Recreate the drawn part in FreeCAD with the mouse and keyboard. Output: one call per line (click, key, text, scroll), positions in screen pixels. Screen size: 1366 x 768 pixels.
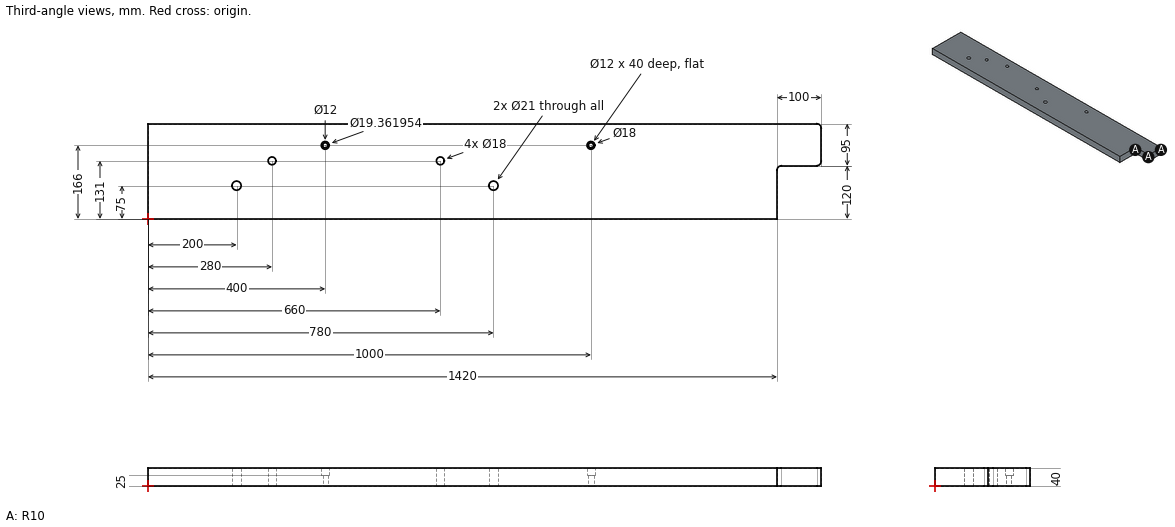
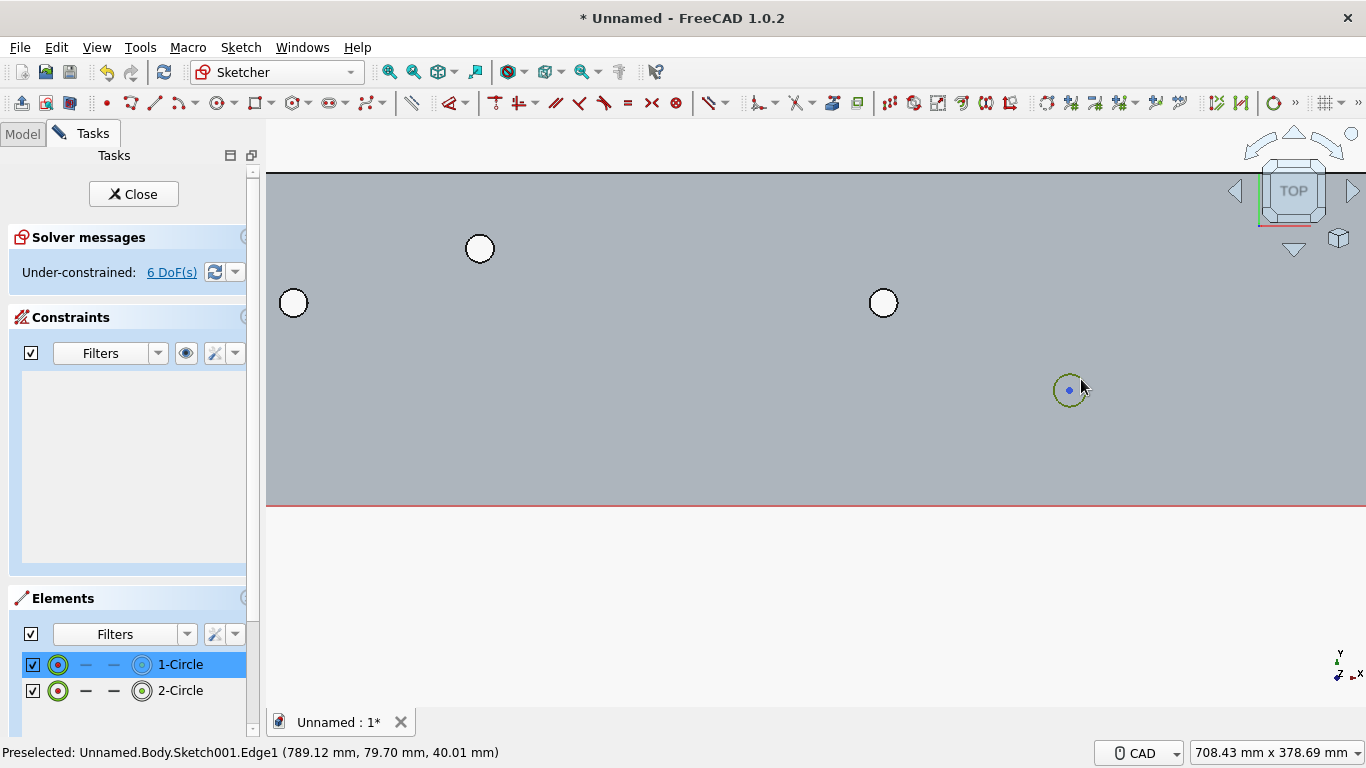
scroll(1082, 380, down, 3)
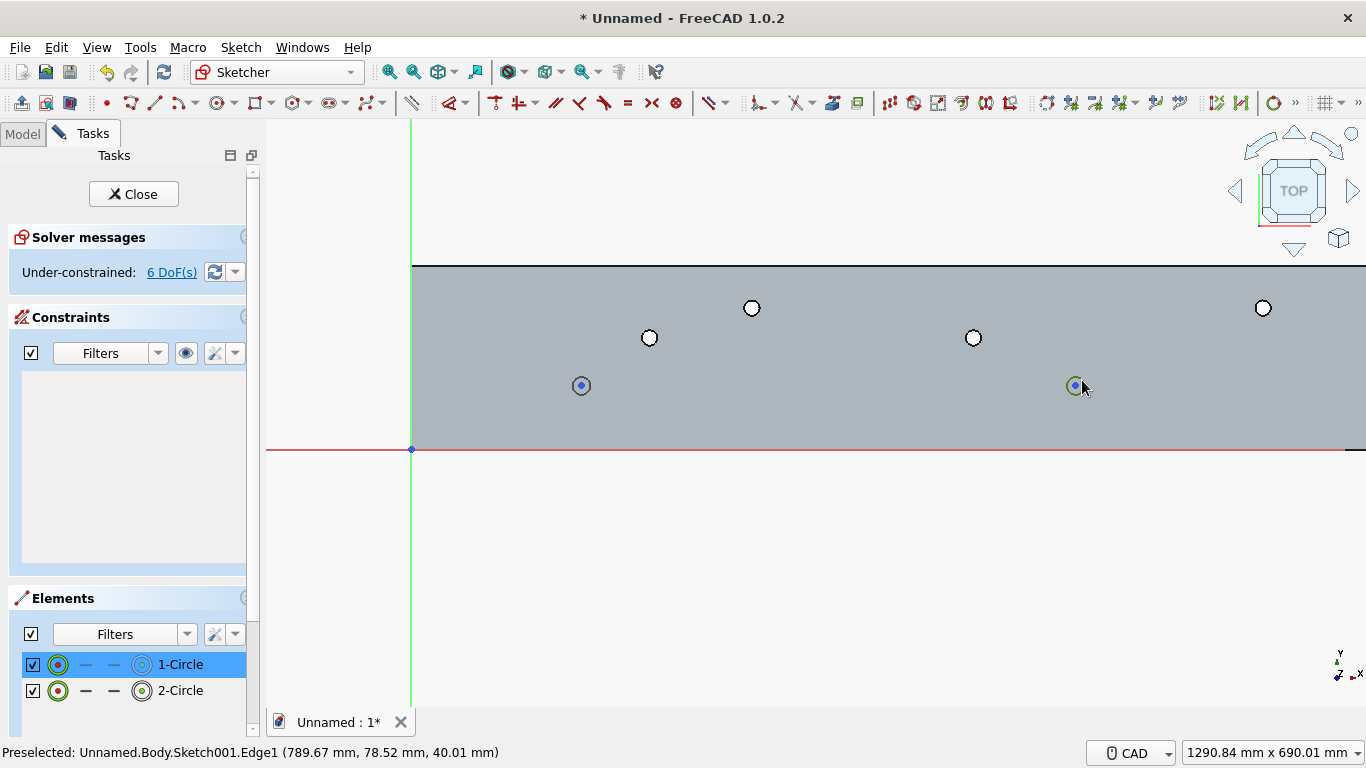
scroll(588, 380, up, 3)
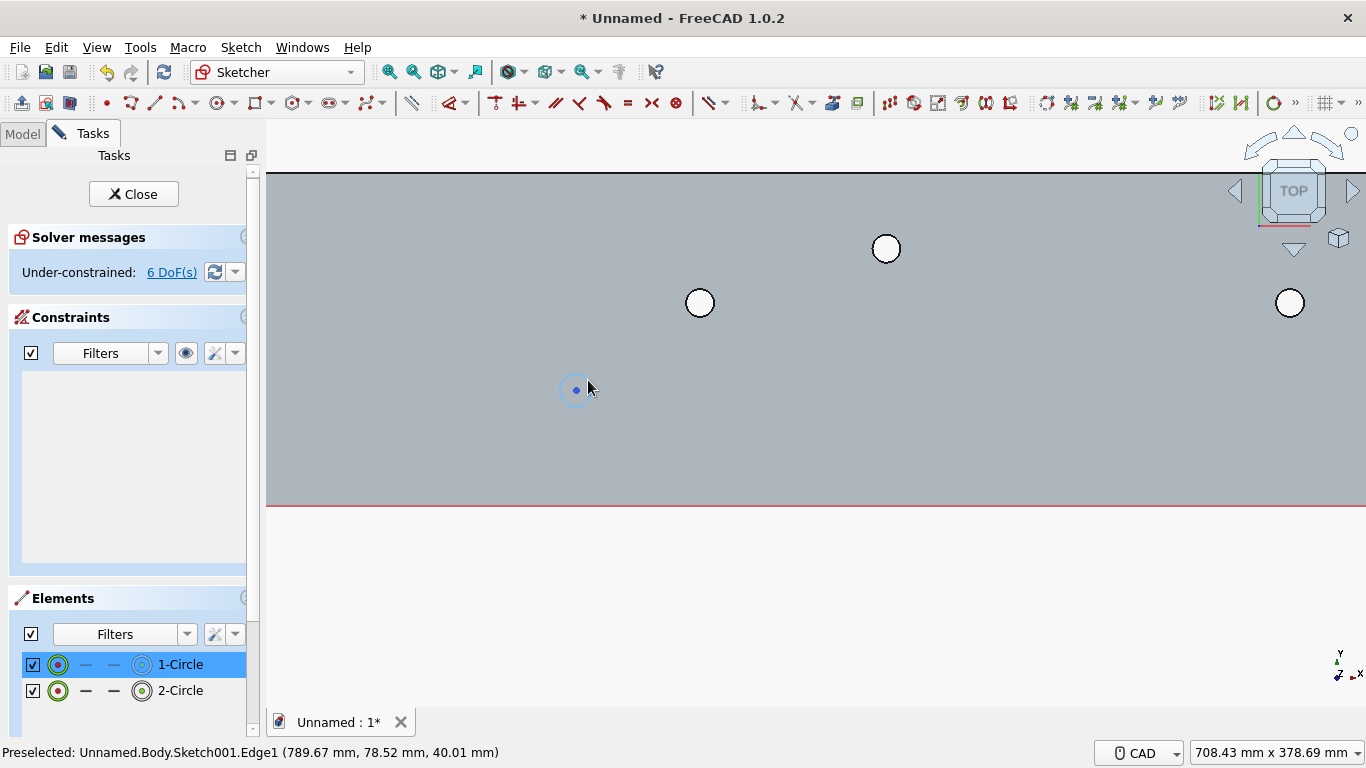
click(587, 379)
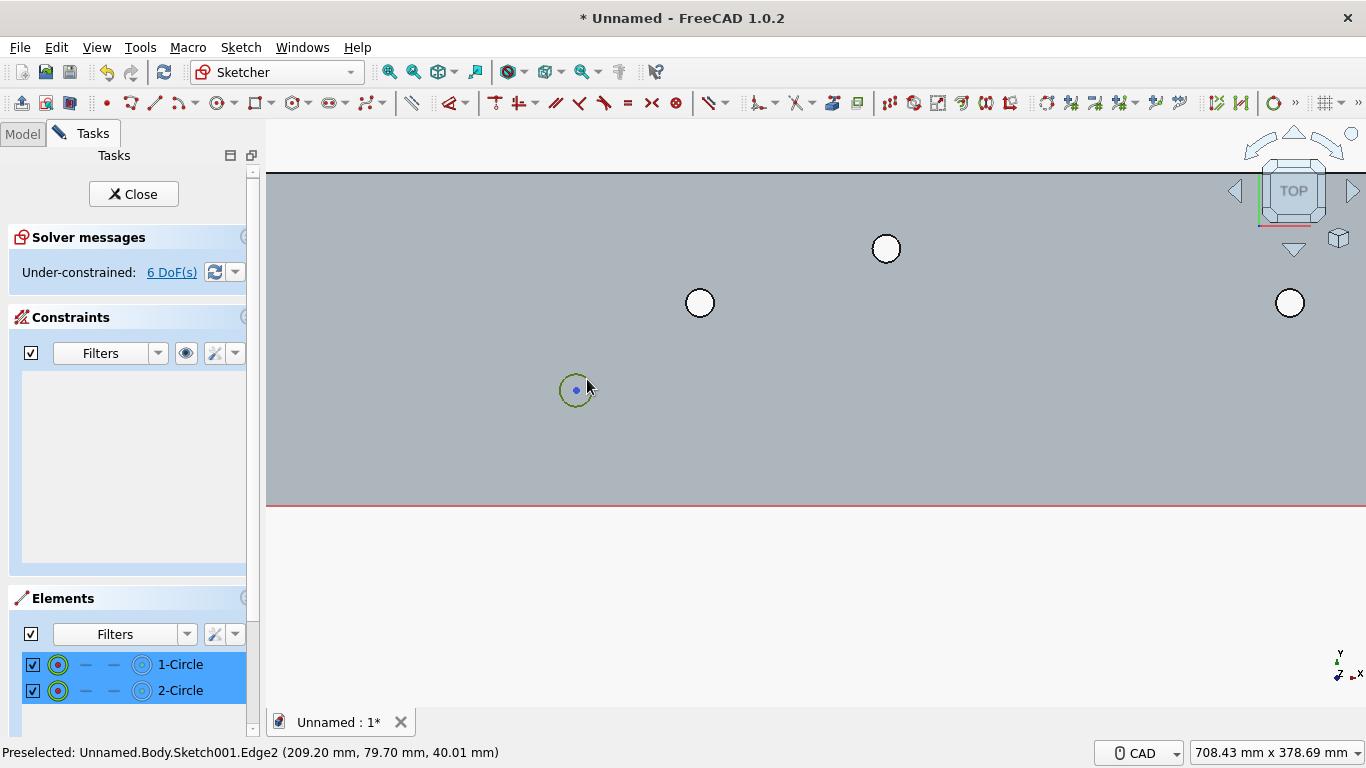
key(e)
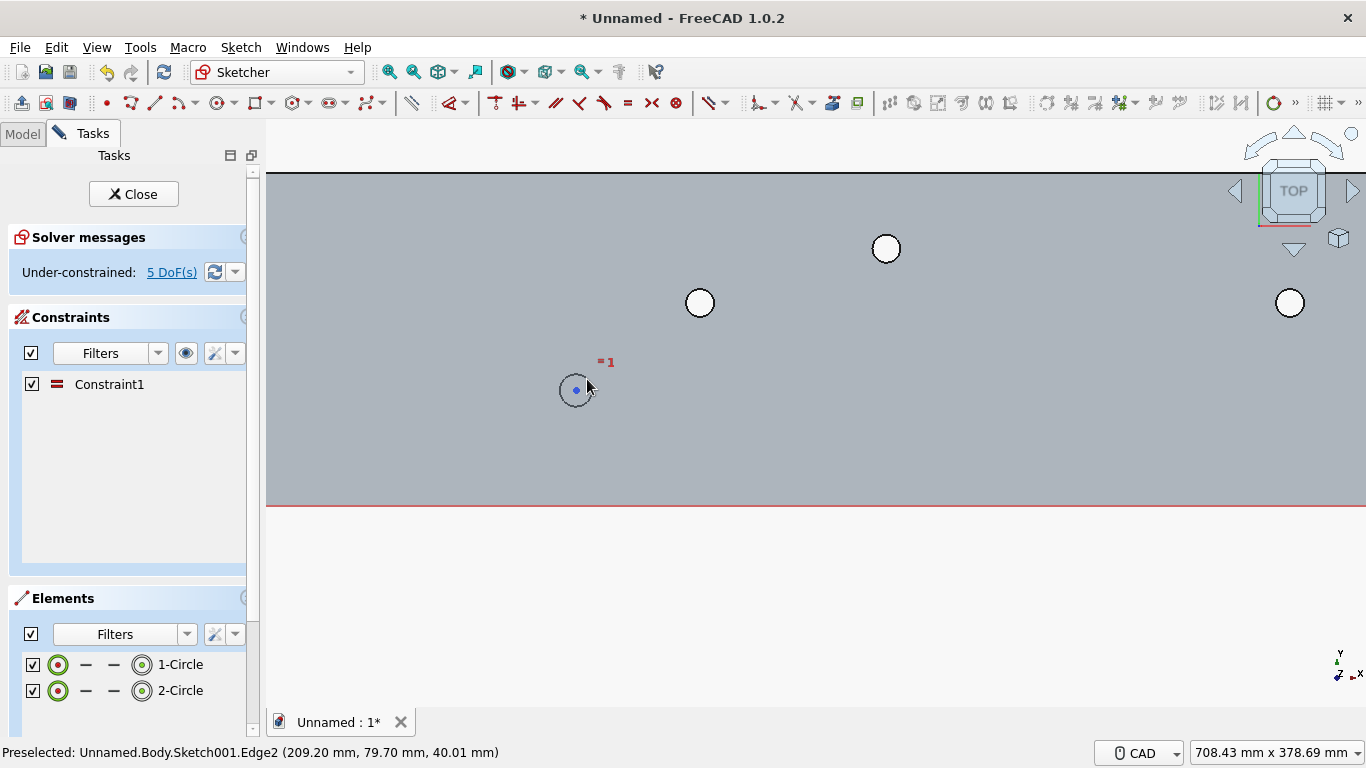
click(450, 104)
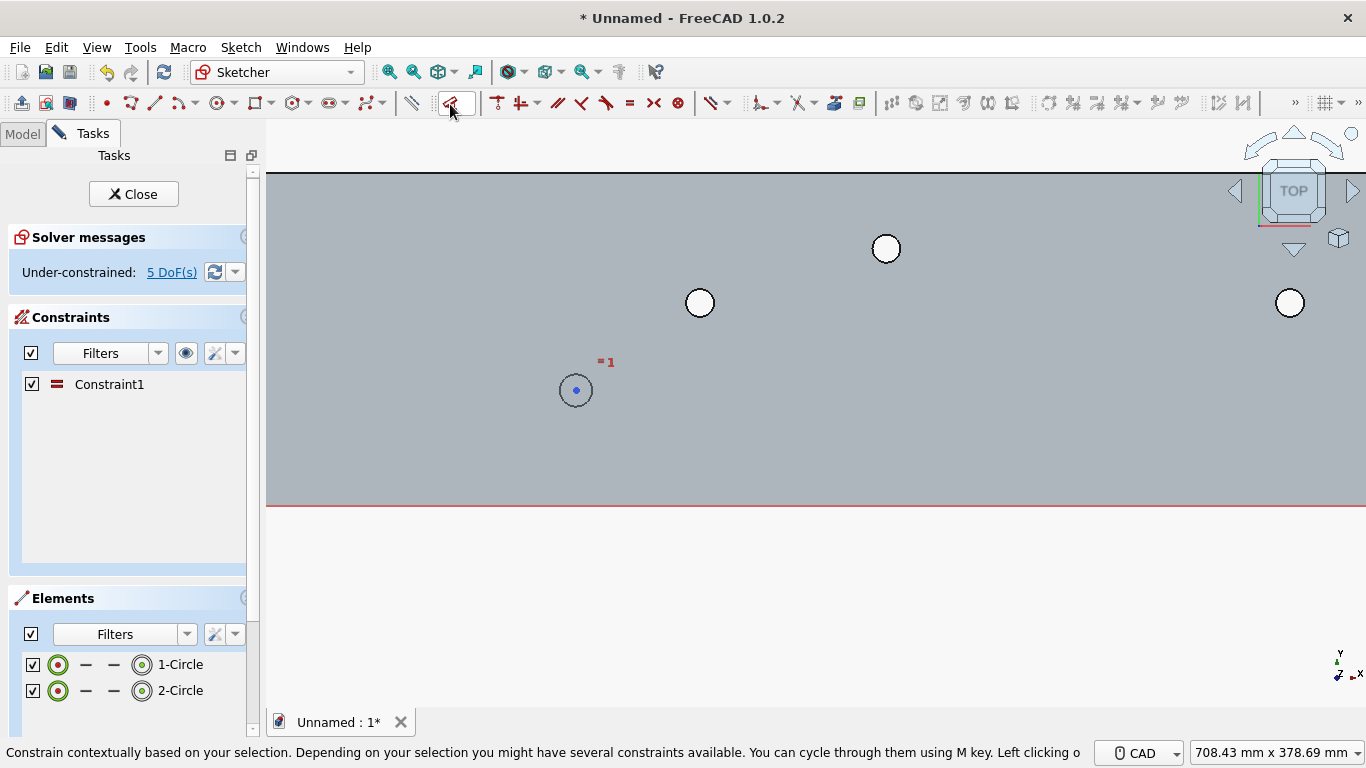
scroll(588, 380, down, 3)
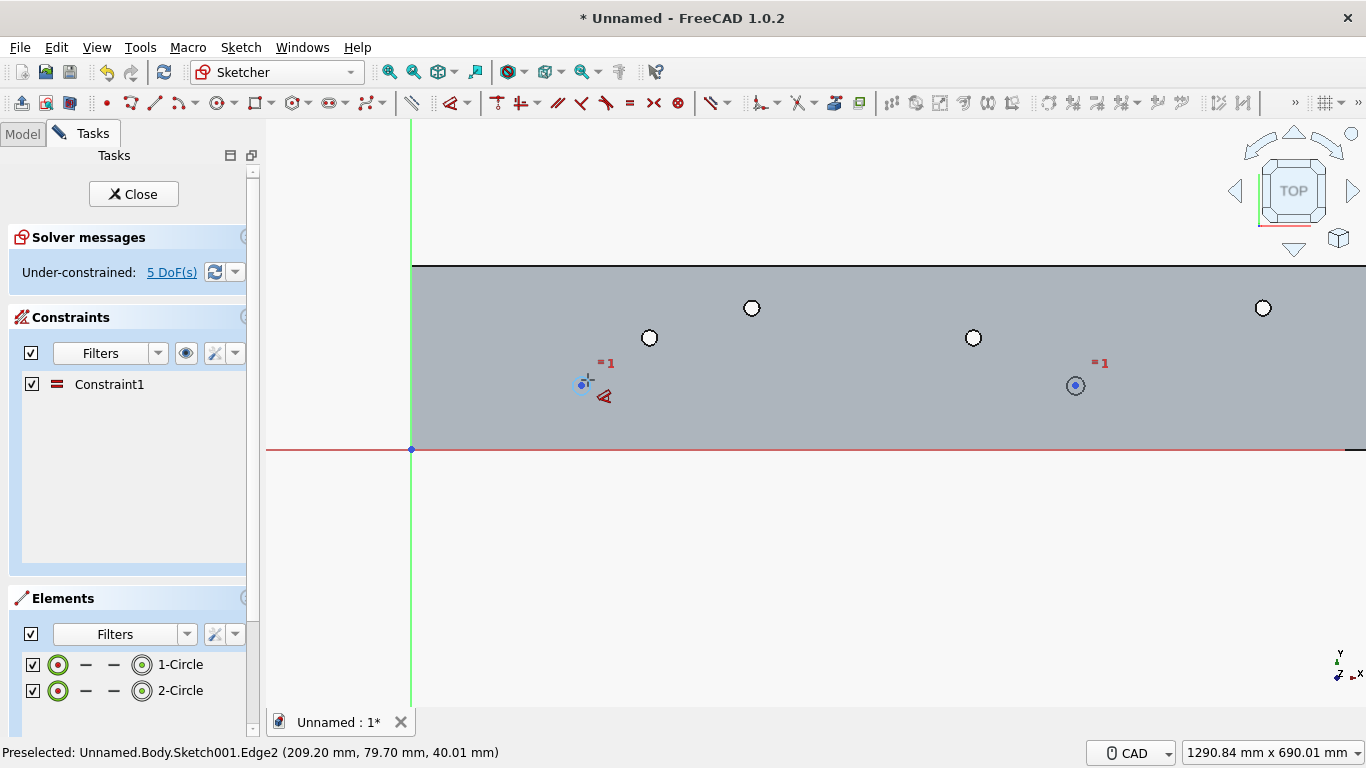
scroll(1082, 380, up, 4)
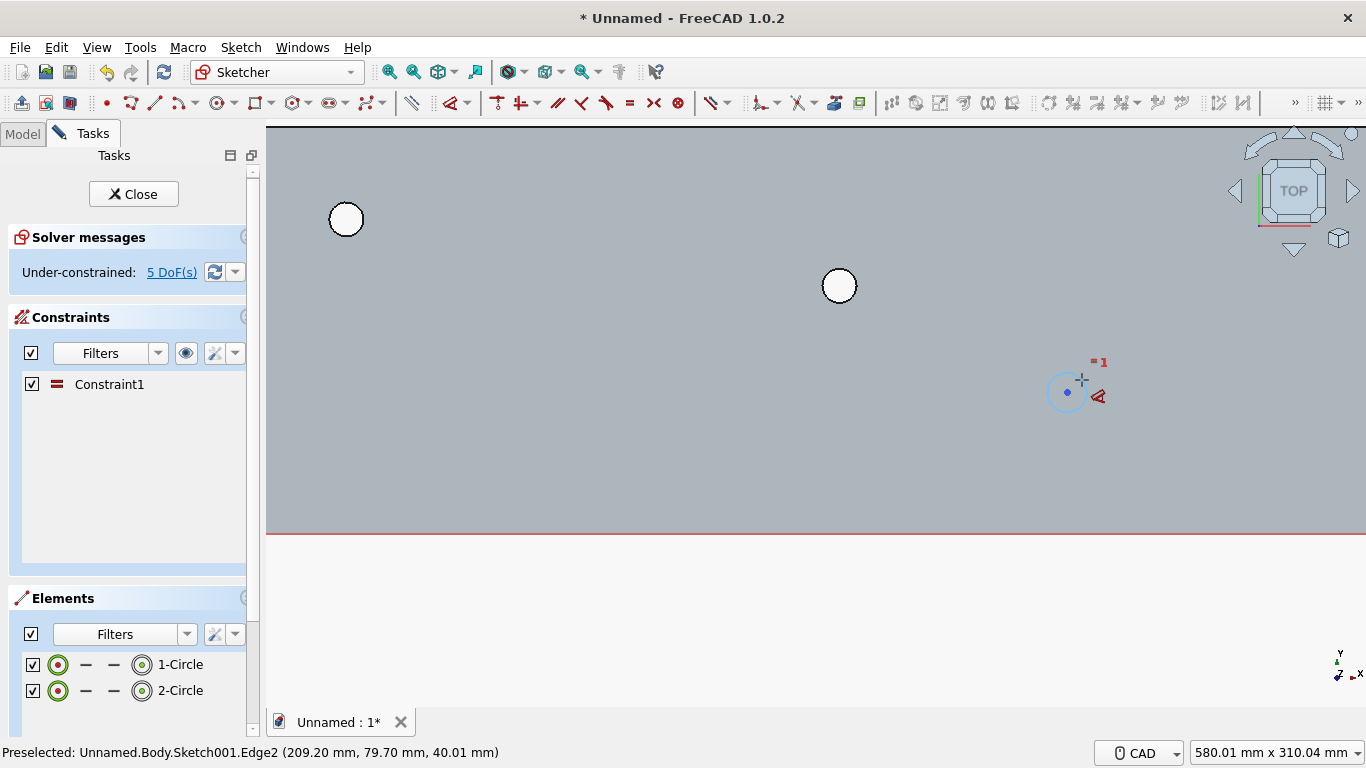
click(1081, 379)
click(1104, 357)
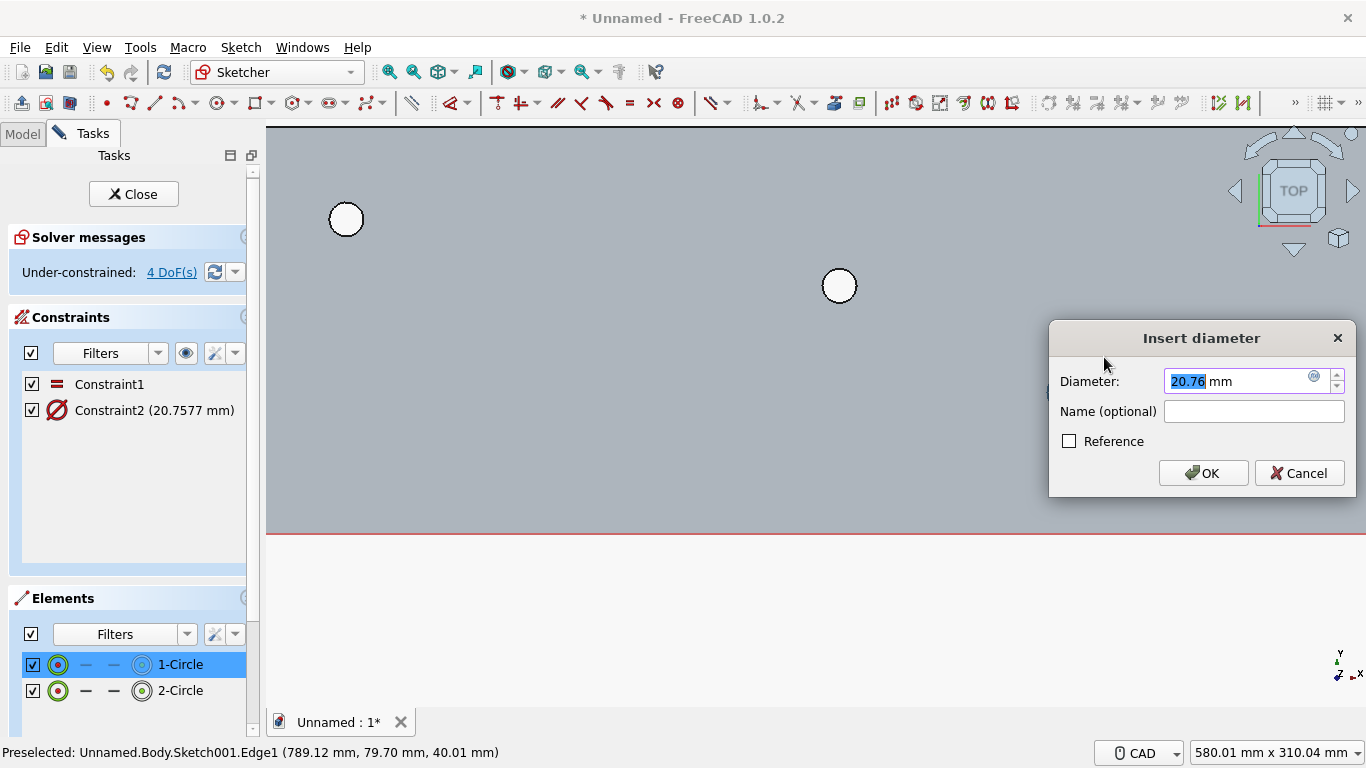
text(21)
key(Return)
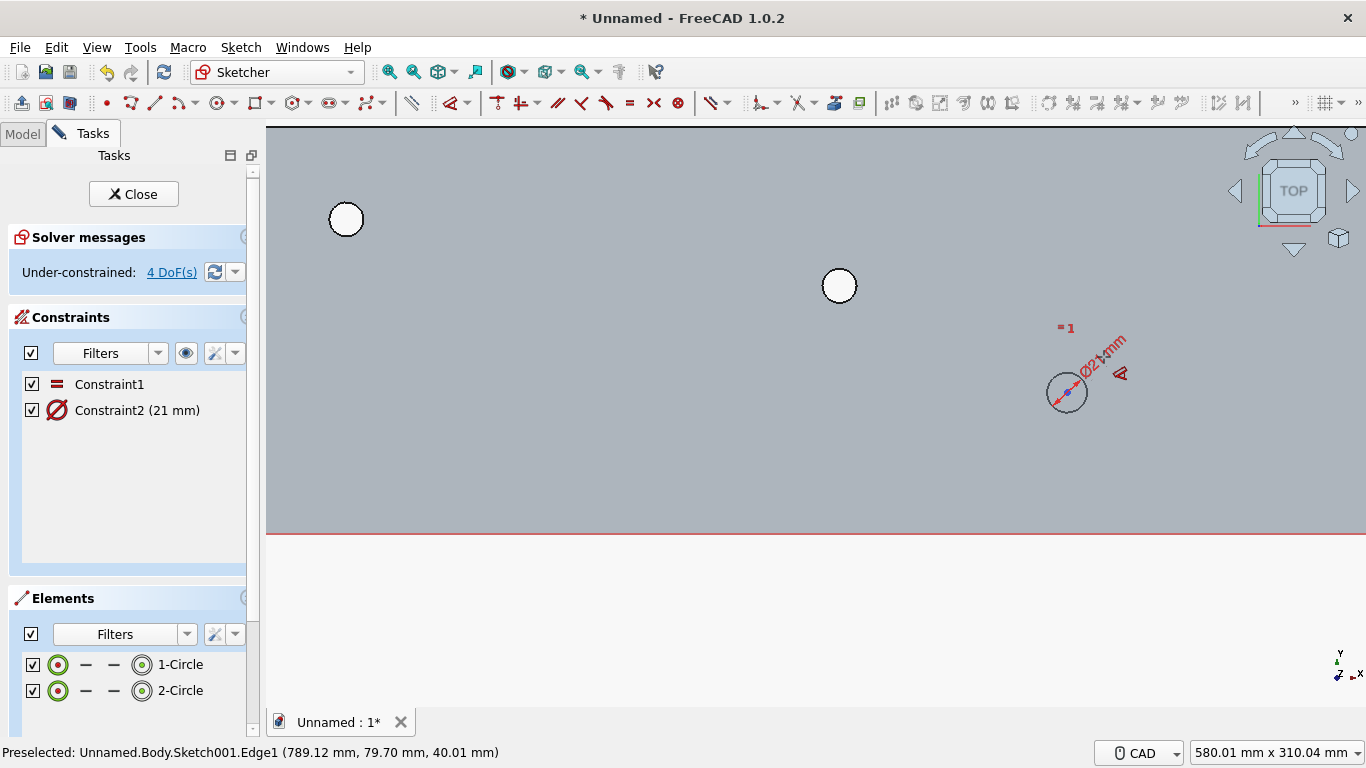
click(1067, 393)
click(1101, 463)